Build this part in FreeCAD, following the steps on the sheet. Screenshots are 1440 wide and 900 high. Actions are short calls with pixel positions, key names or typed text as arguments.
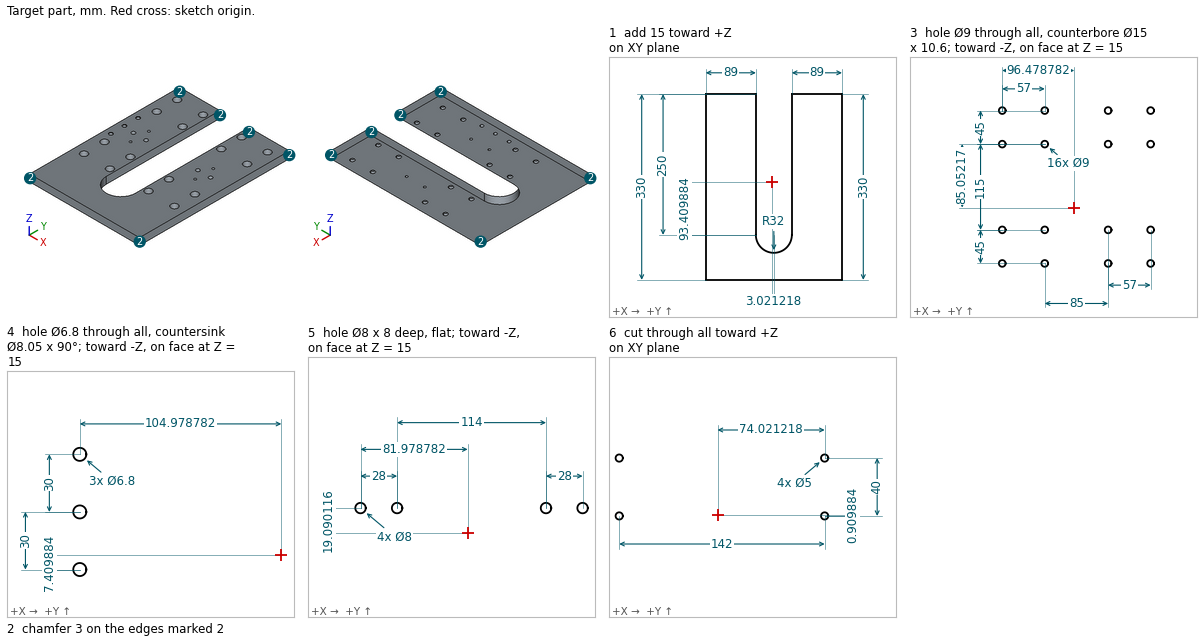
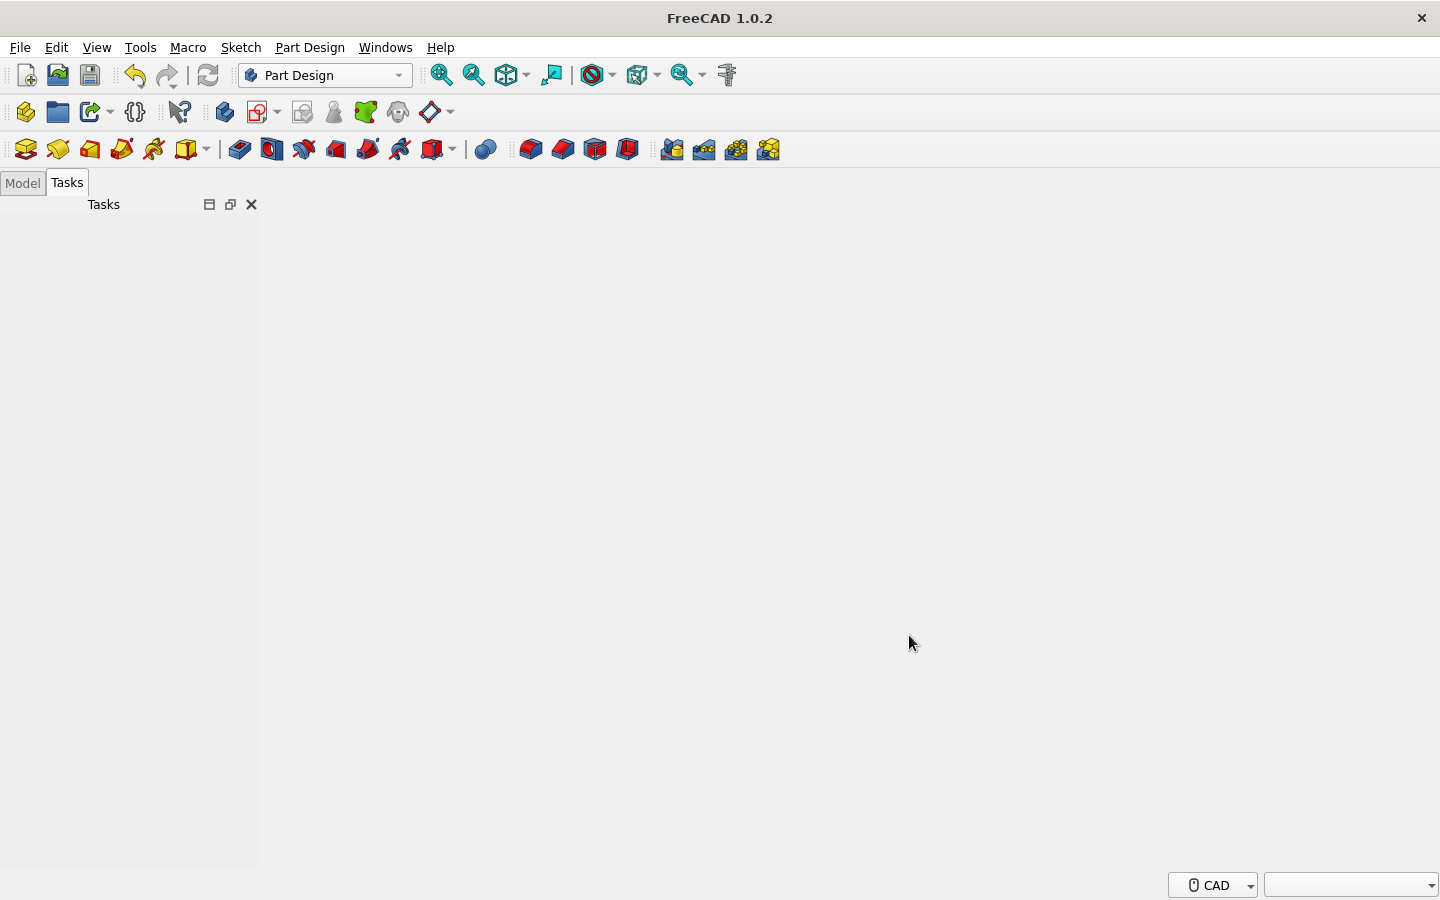
click(26, 76)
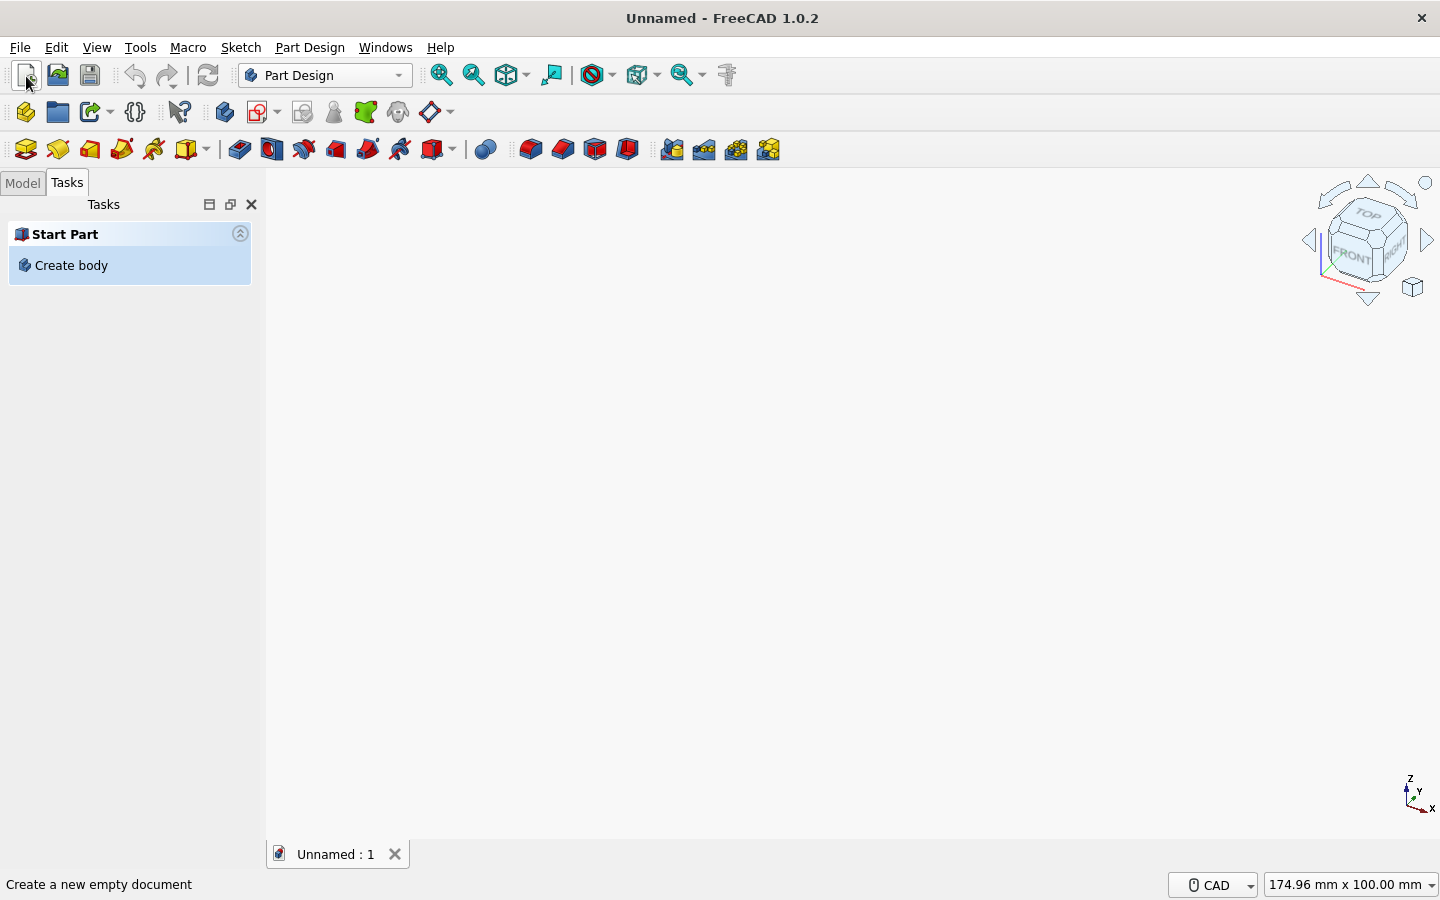
click(258, 112)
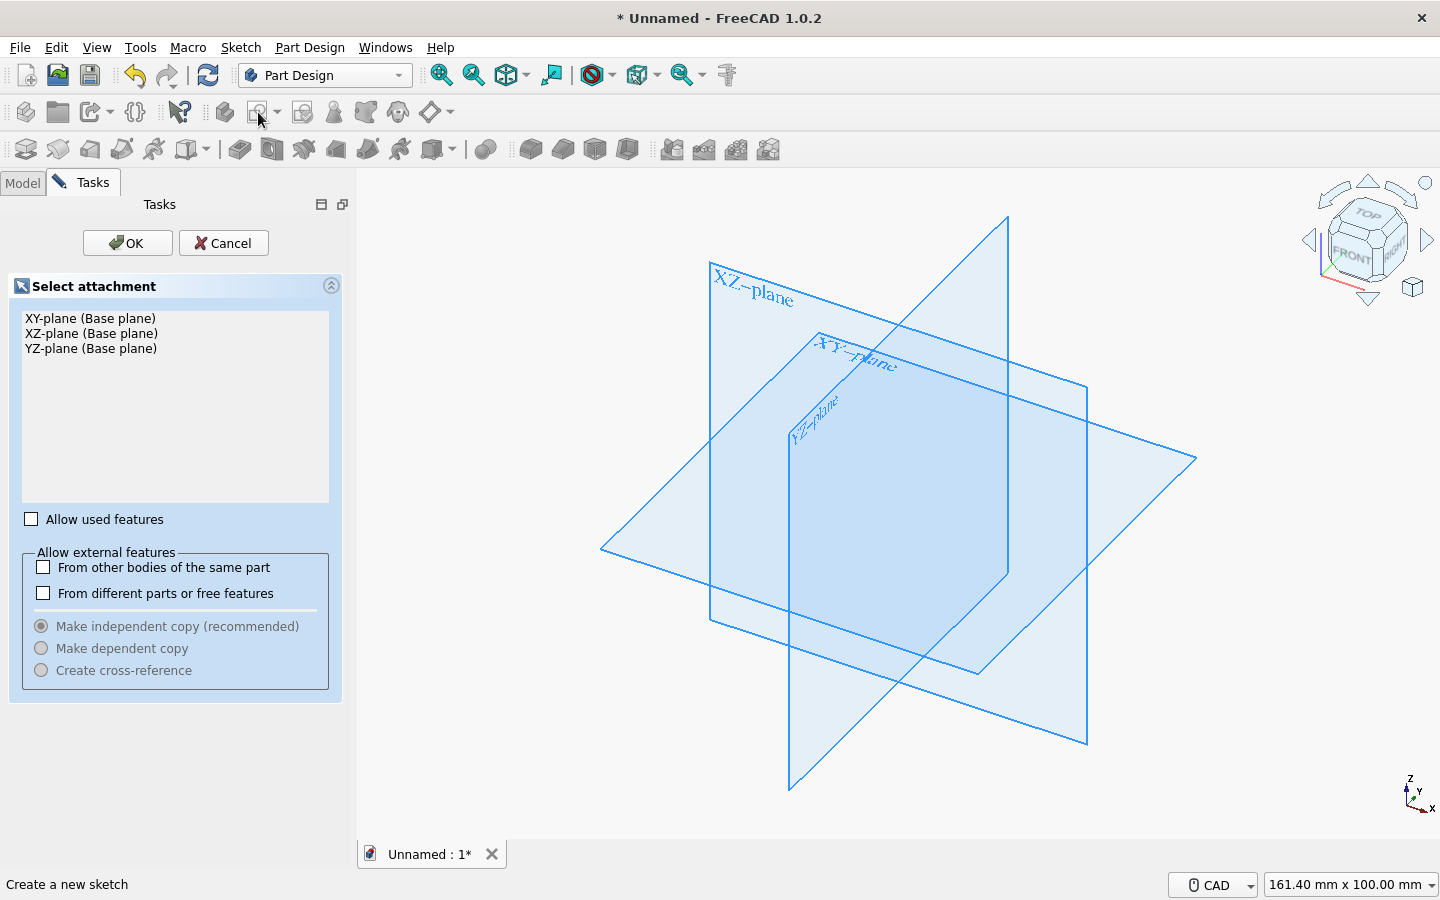
click(82, 318)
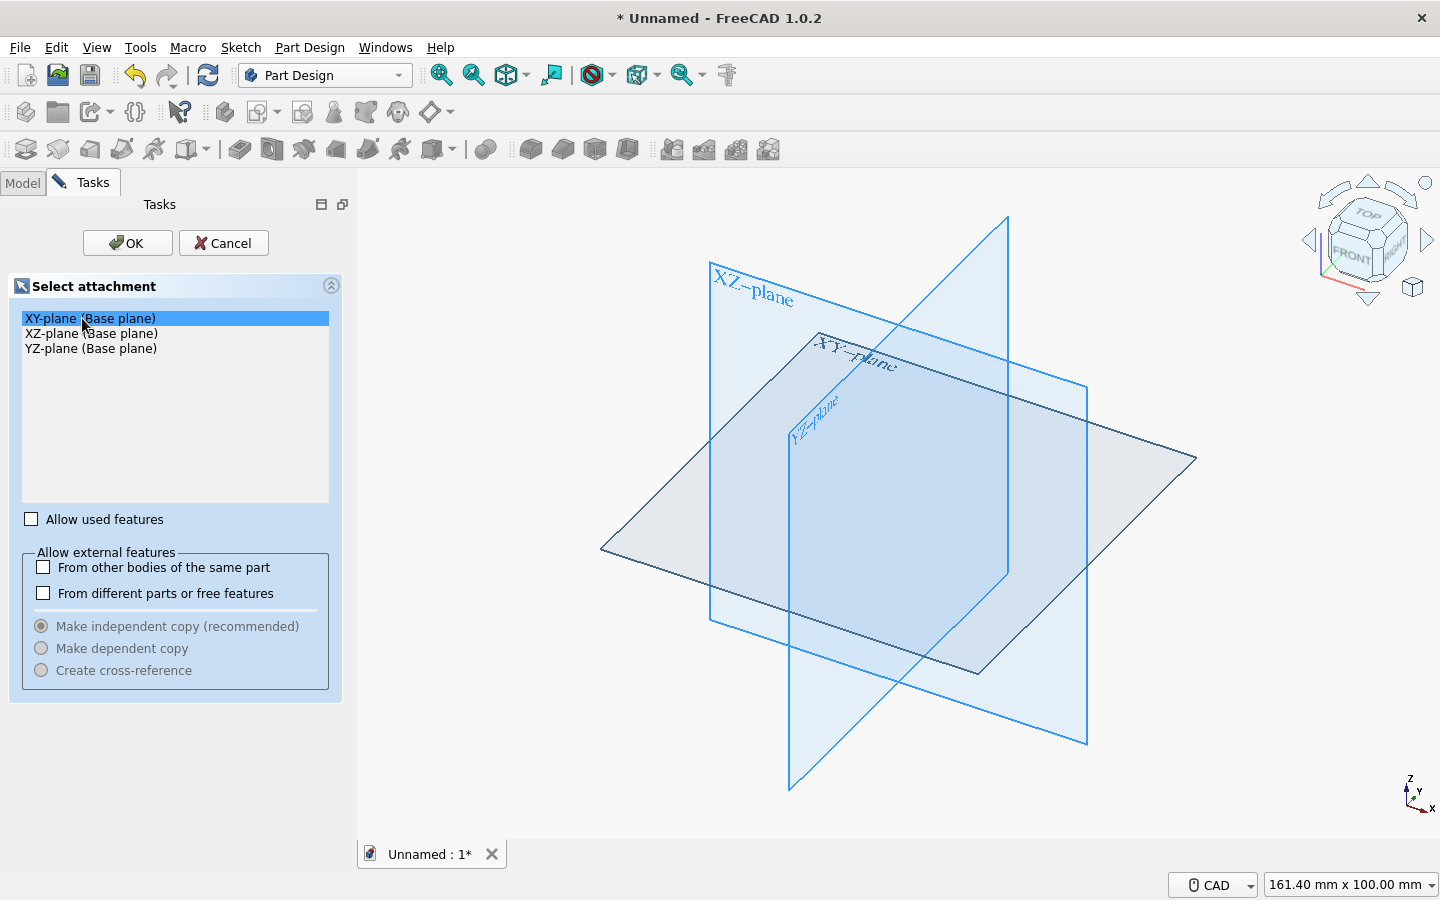
click(128, 243)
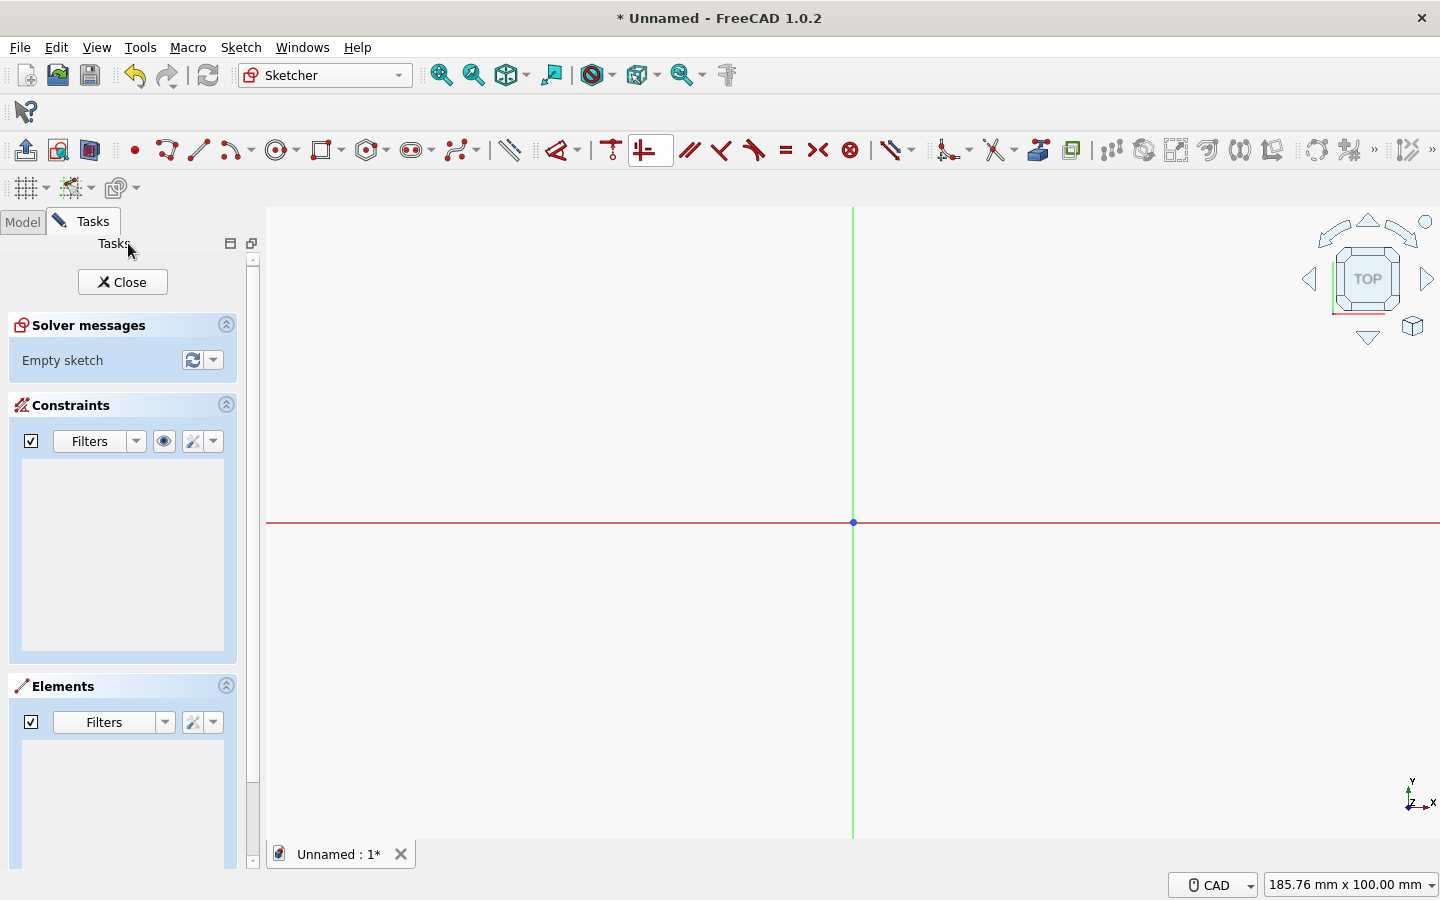
scroll(762, 510, down, 8)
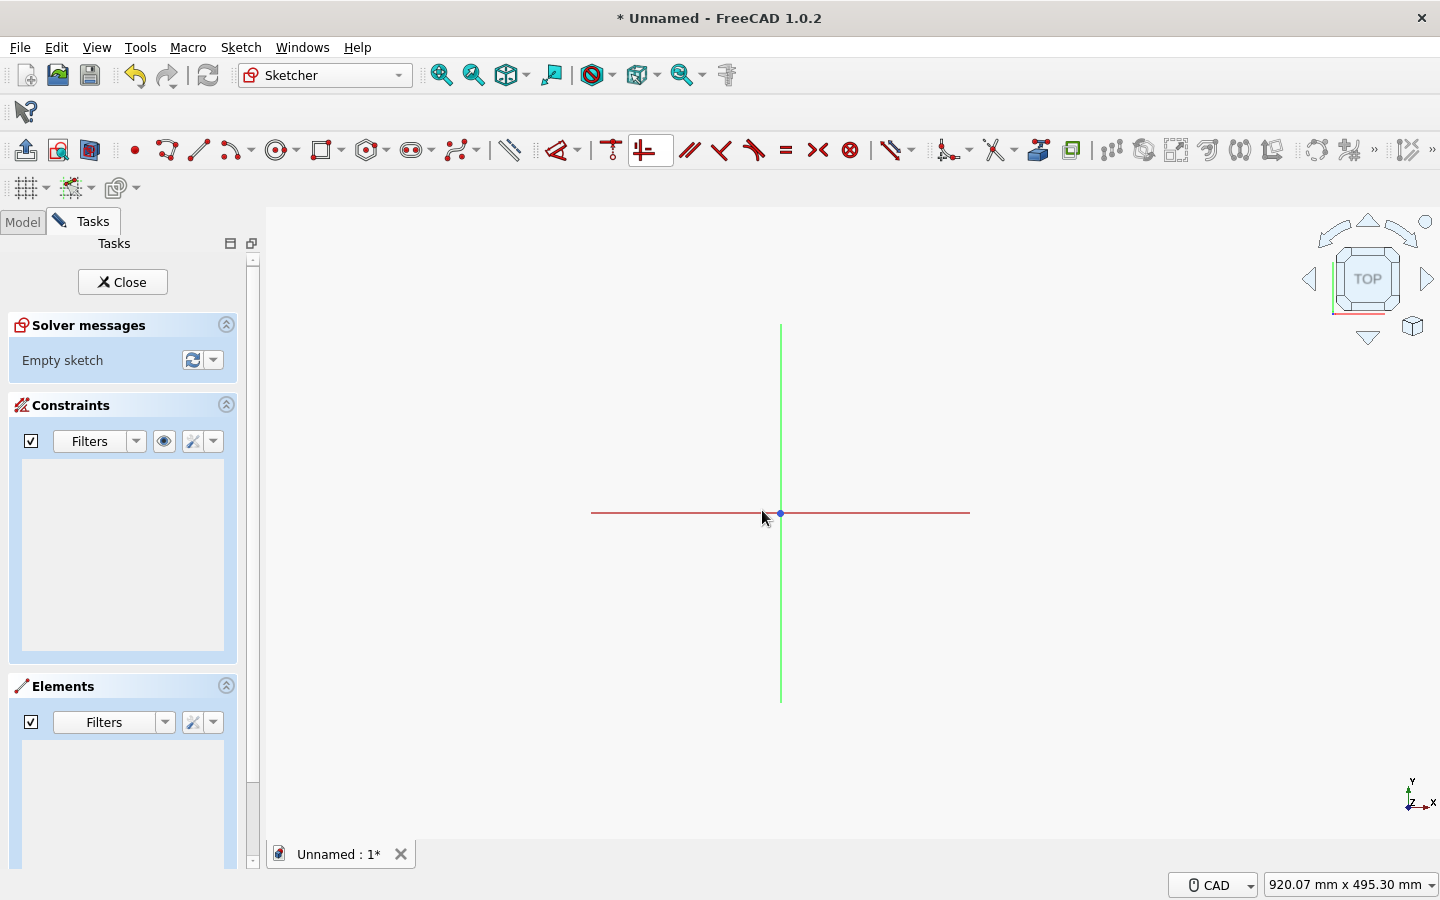
click(168, 150)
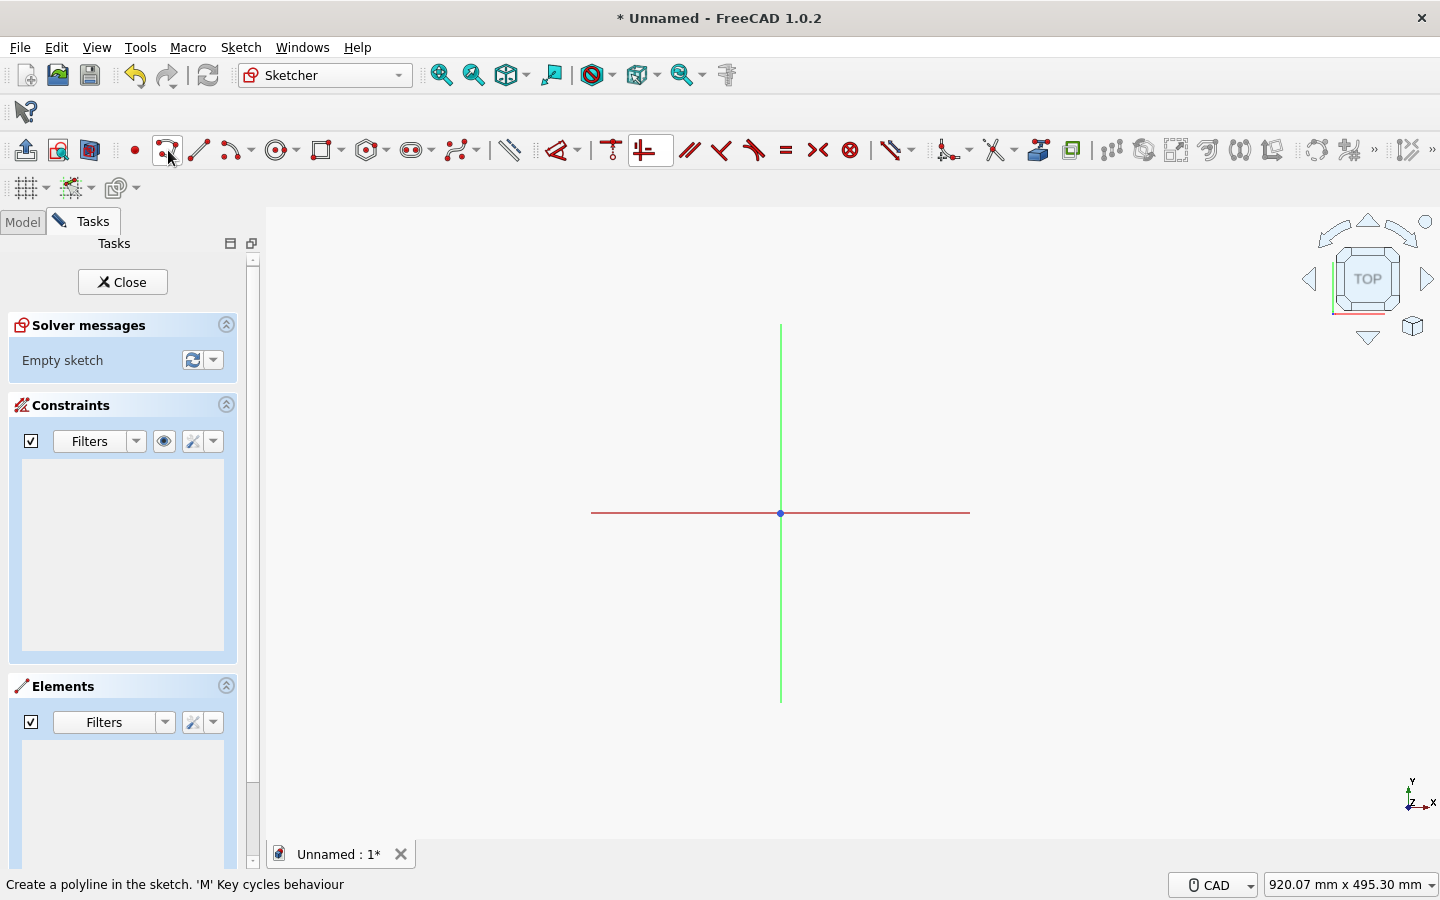
click(744, 632)
click(744, 313)
click(630, 313)
click(630, 734)
click(939, 734)
click(939, 313)
click(825, 313)
click(825, 632)
right_click(825, 632)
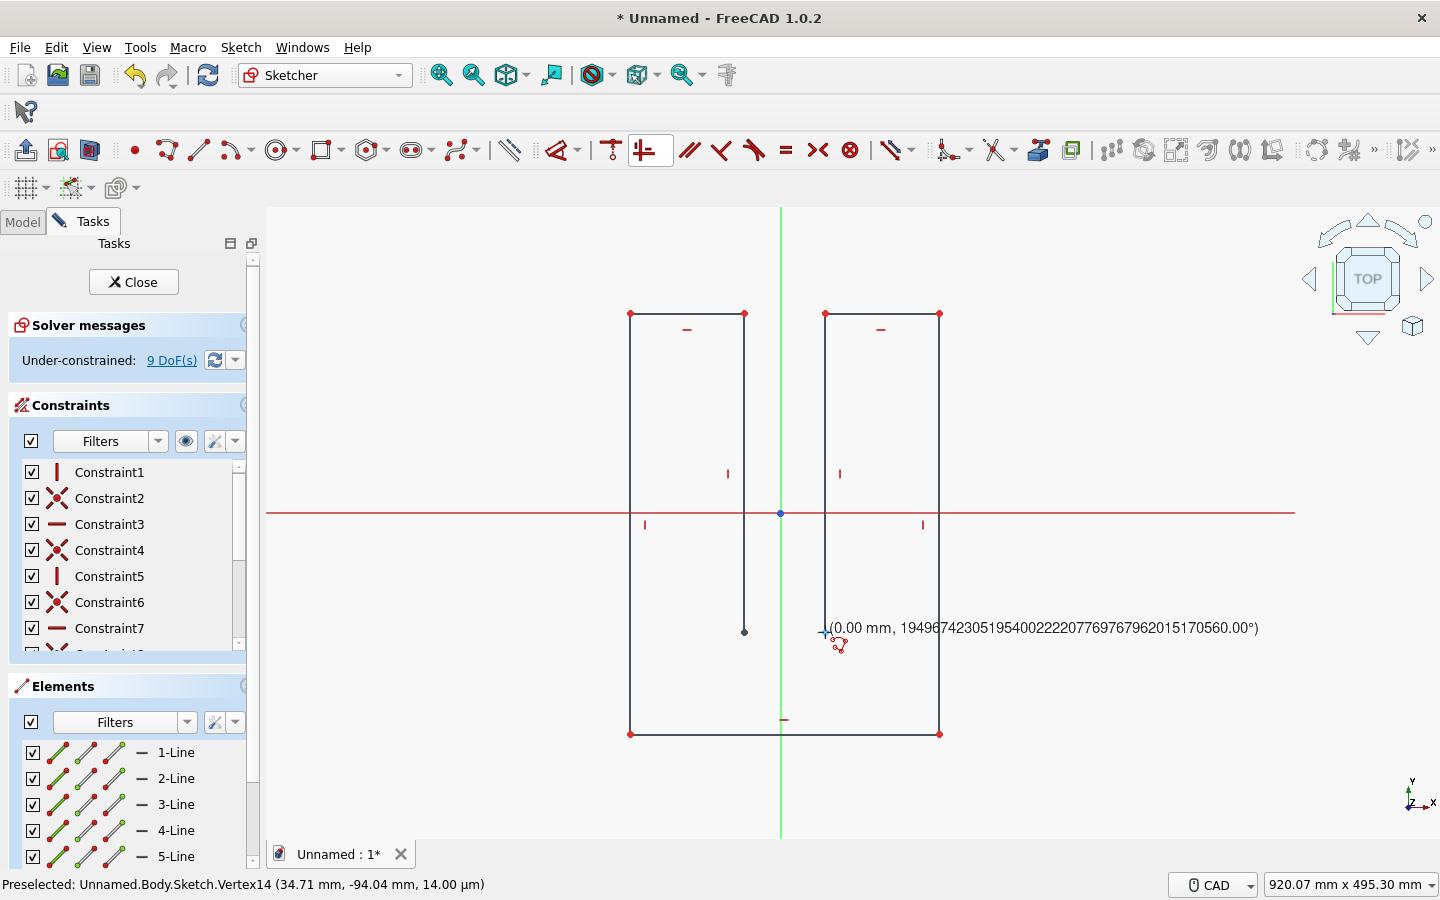
click(254, 150)